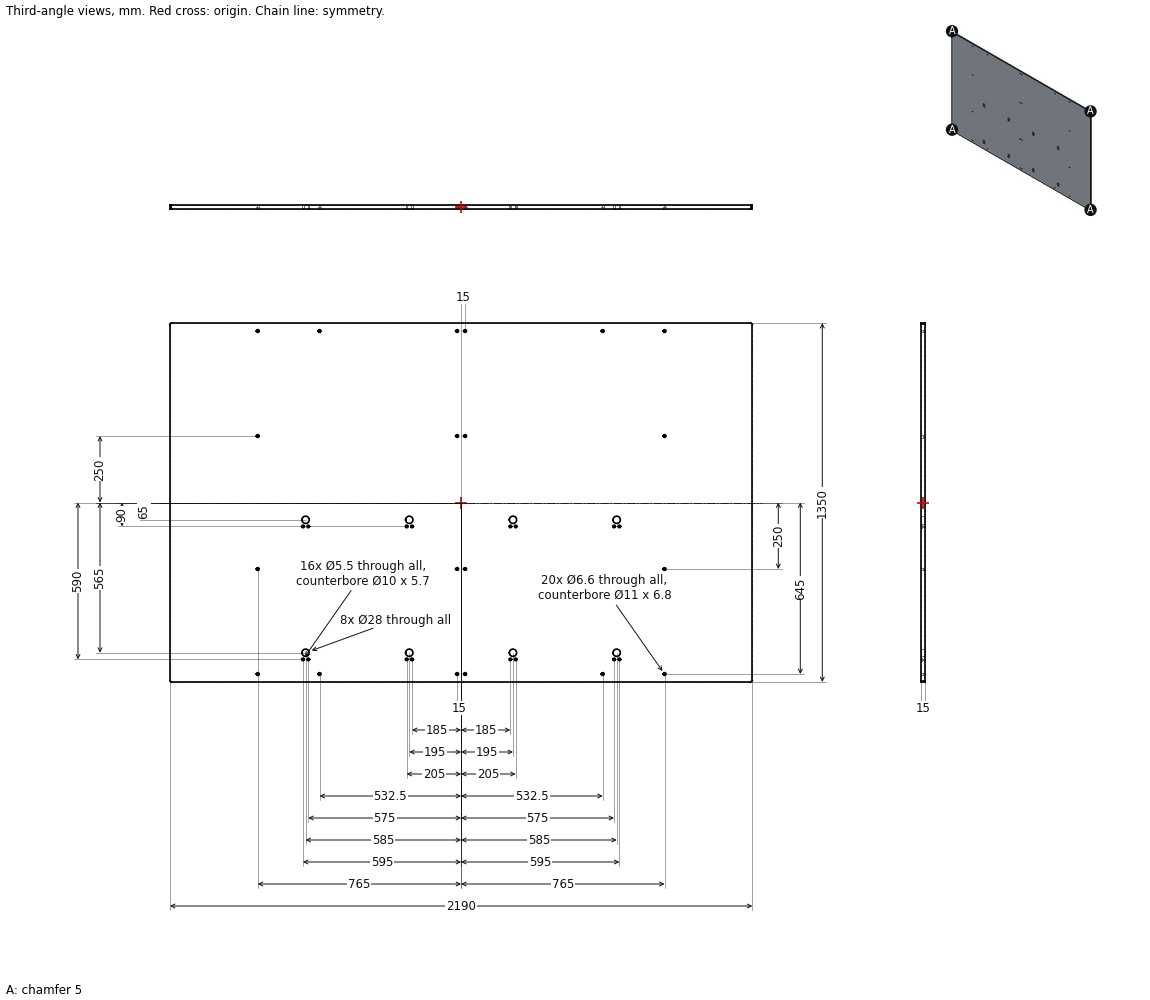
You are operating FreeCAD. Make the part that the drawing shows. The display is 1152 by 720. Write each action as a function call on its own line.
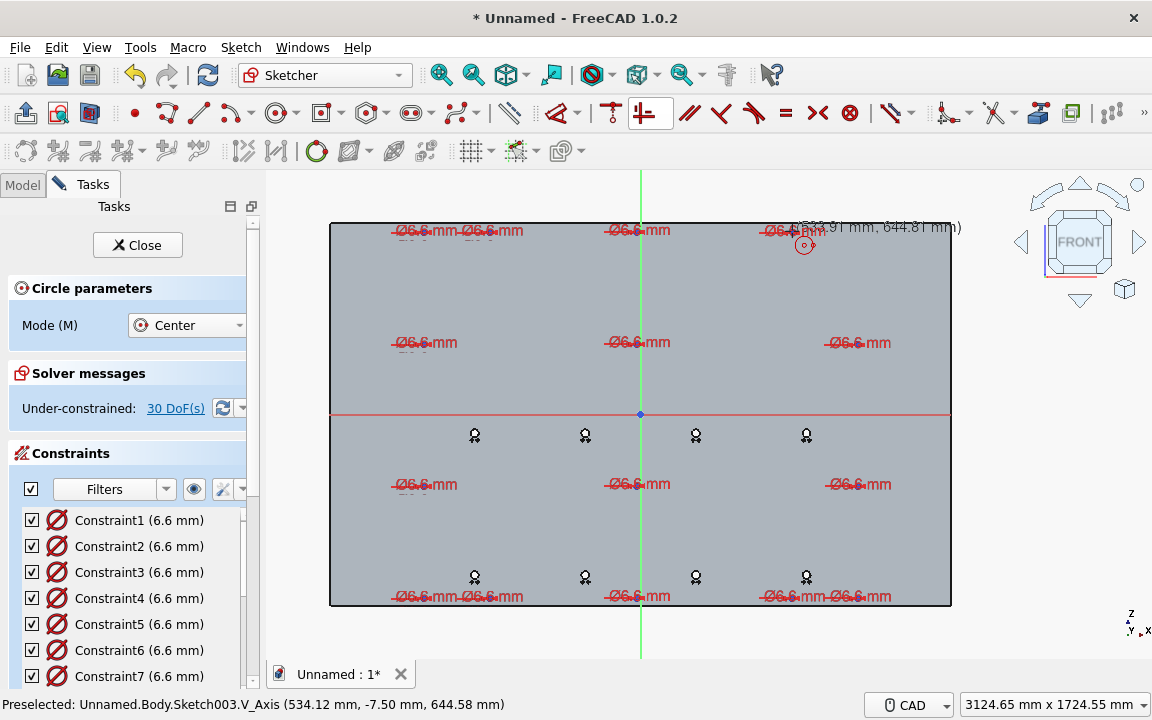
scroll(858, 232, up, 16)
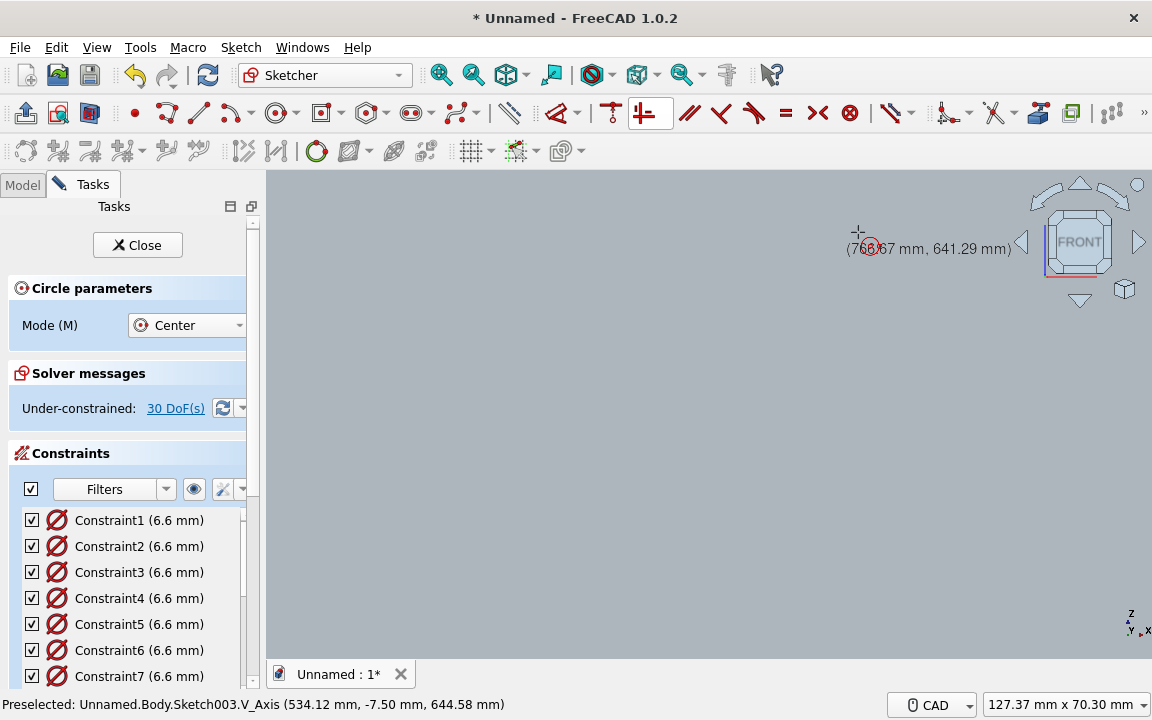
scroll(859, 232, down, 16)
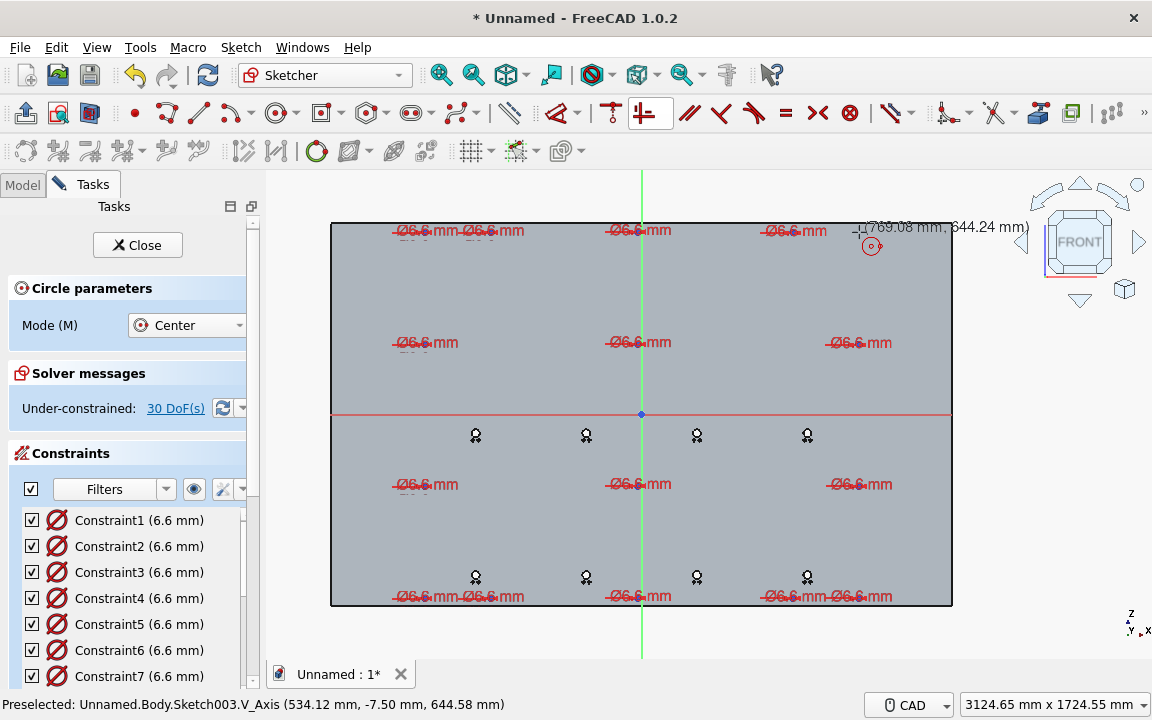
click(858, 232)
move(859, 231)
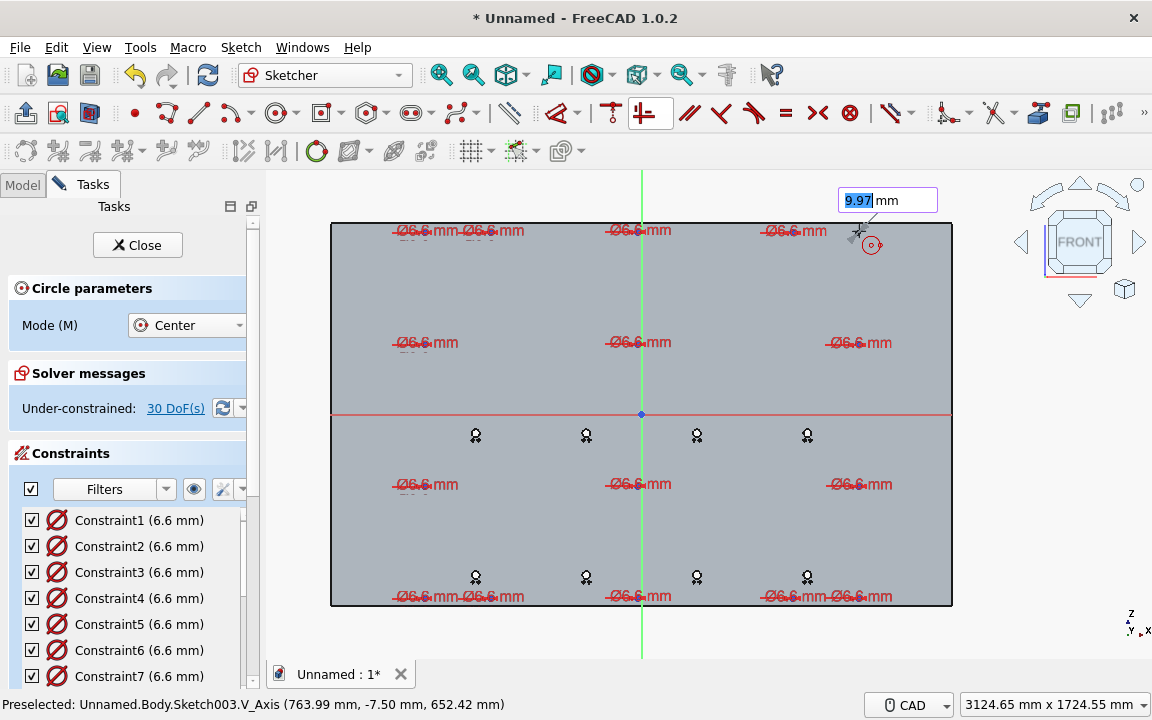
text(6.6)
key(Return)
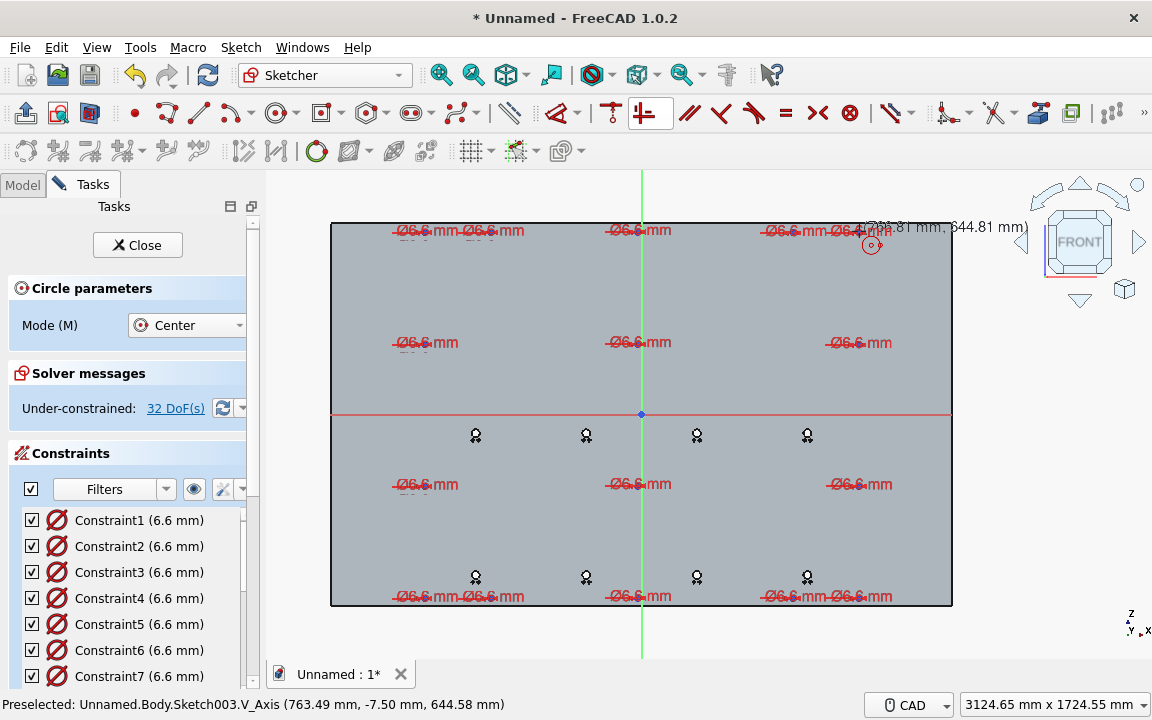
scroll(646, 232, up, 16)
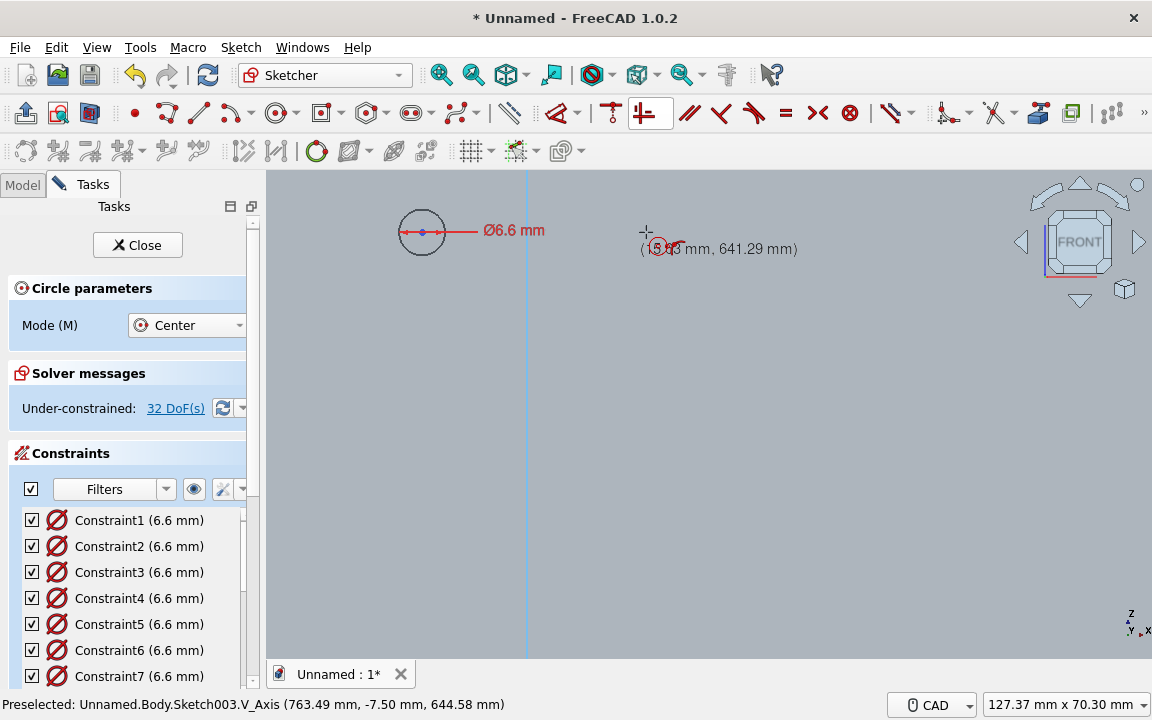
scroll(645, 232, down, 16)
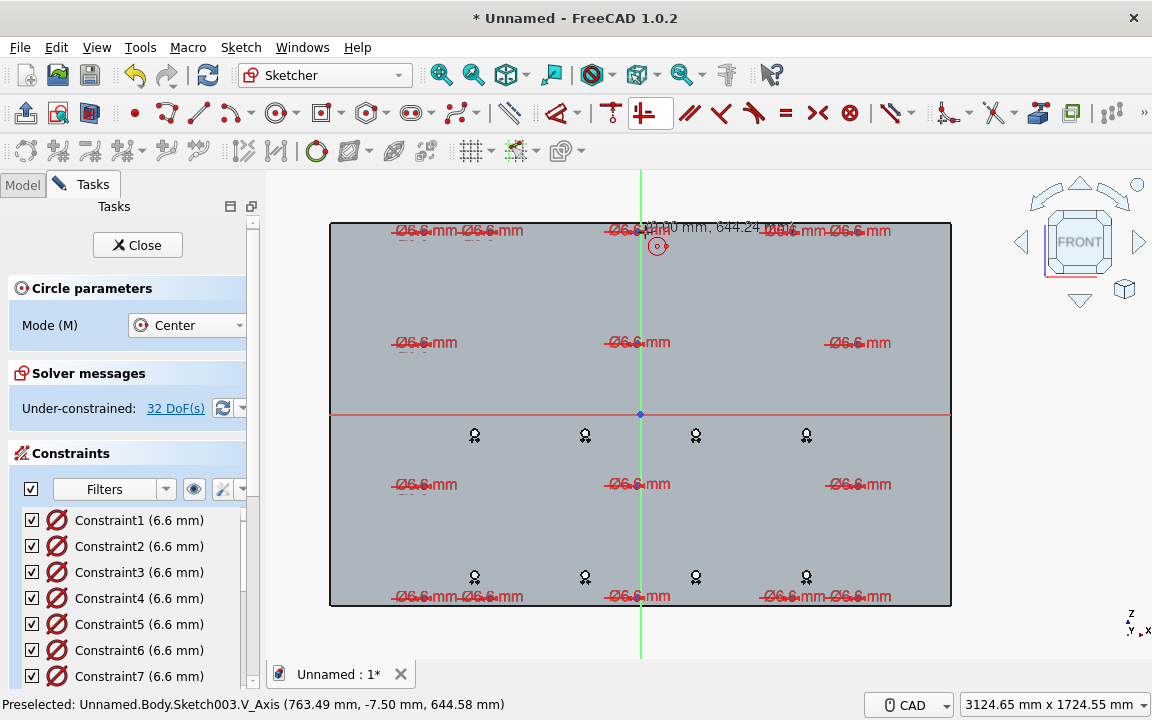
scroll(645, 232, up, 7)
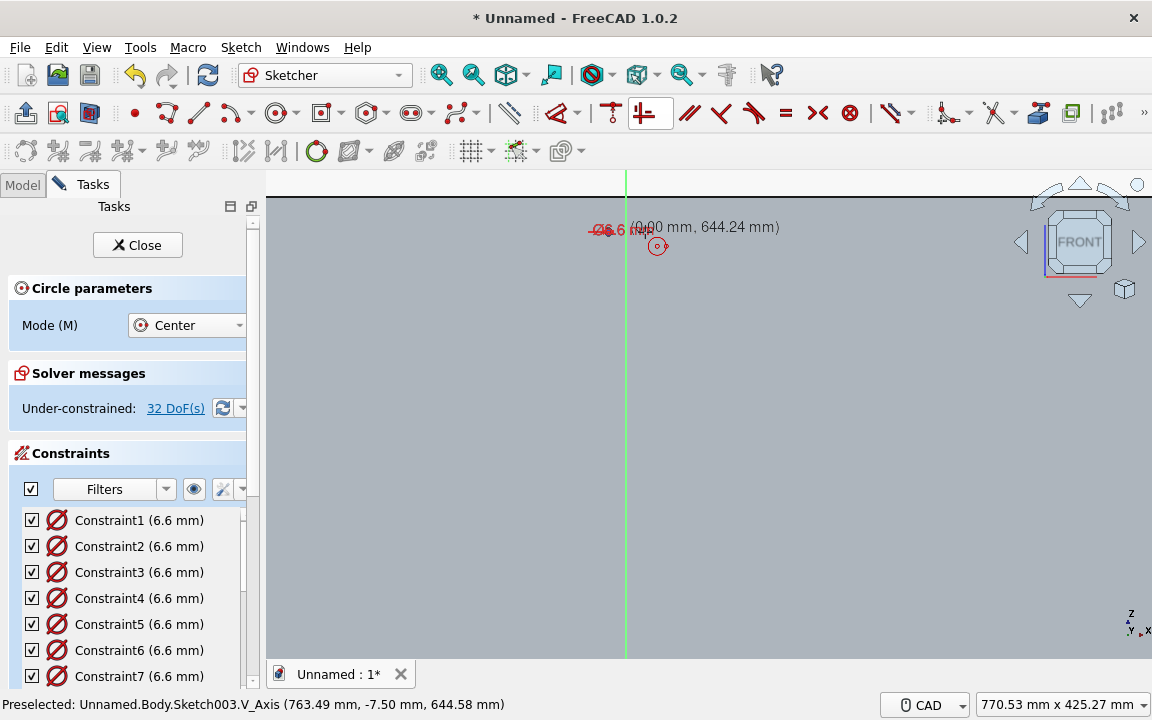
click(643, 231)
move(646, 229)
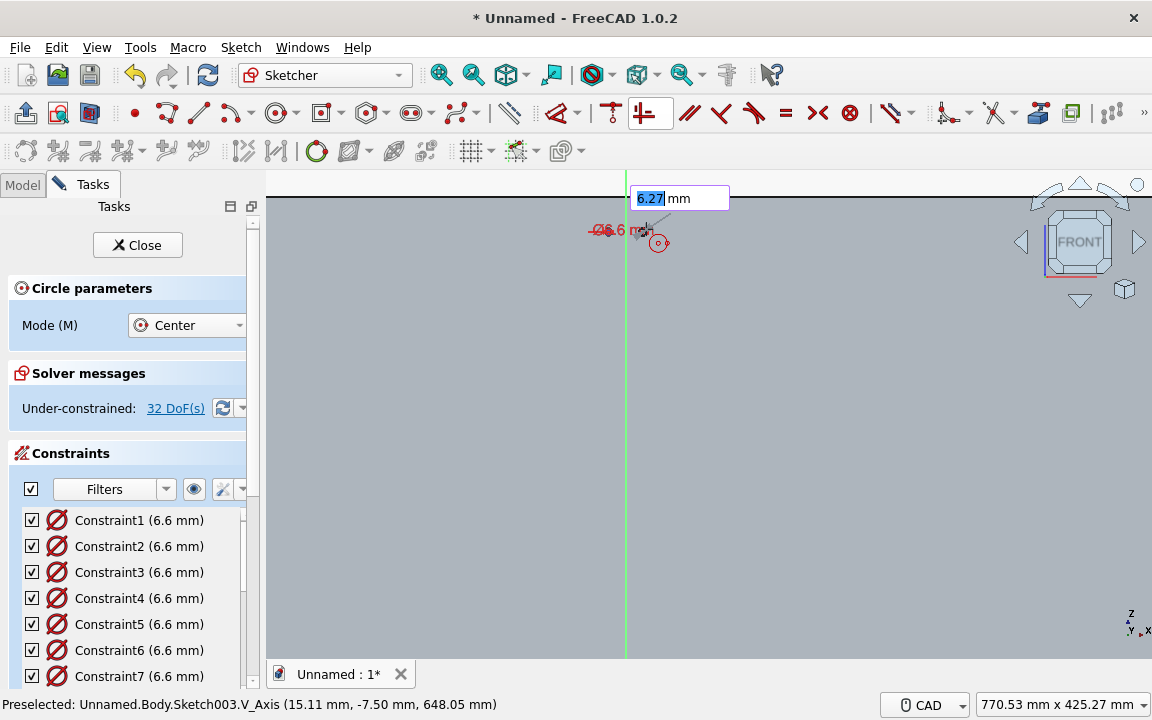
text(6.6)
key(Return)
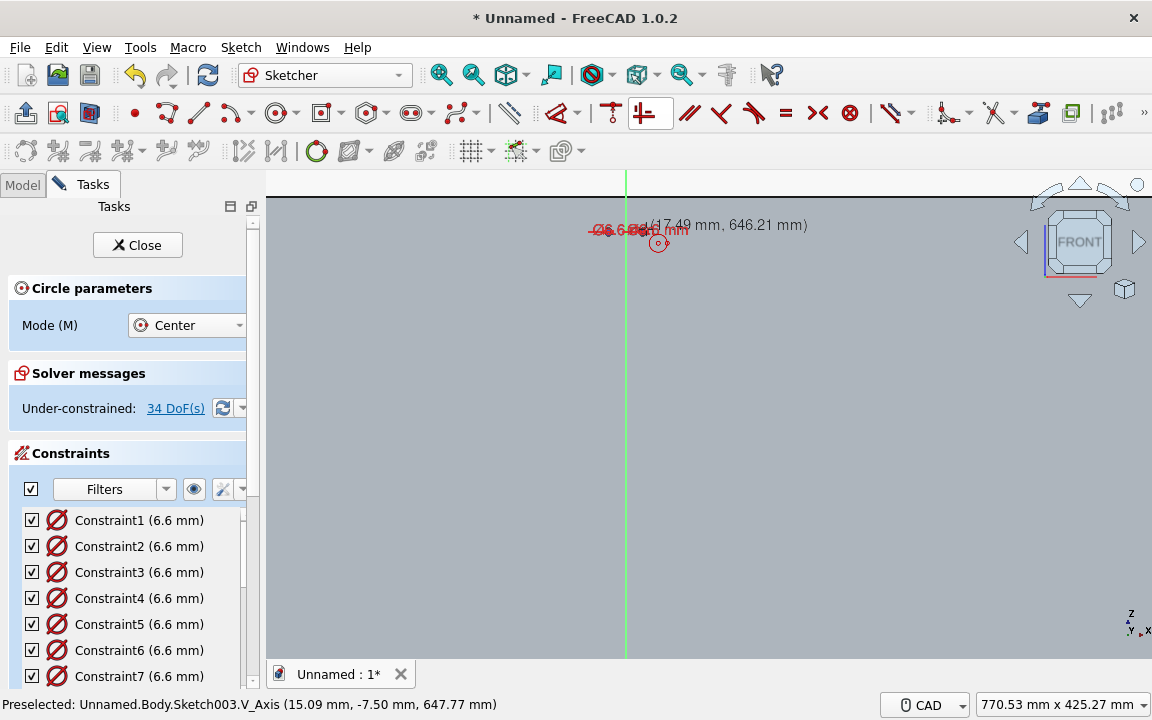
scroll(644, 273, down, 8)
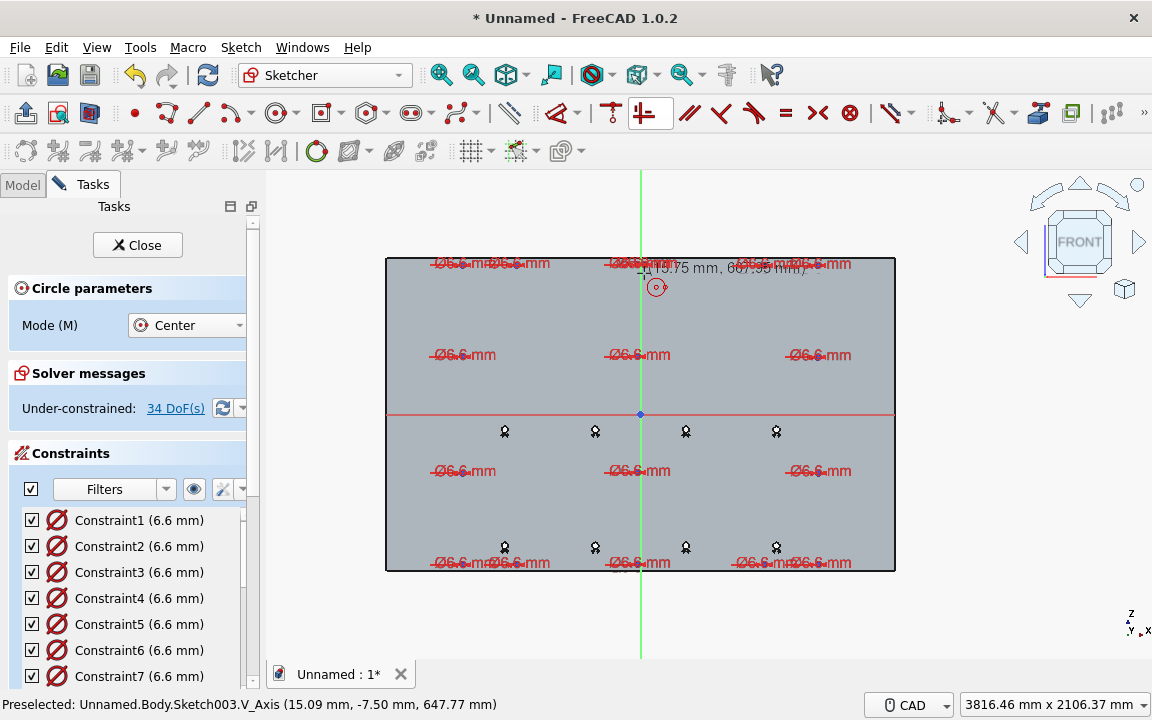
scroll(644, 356, up, 17)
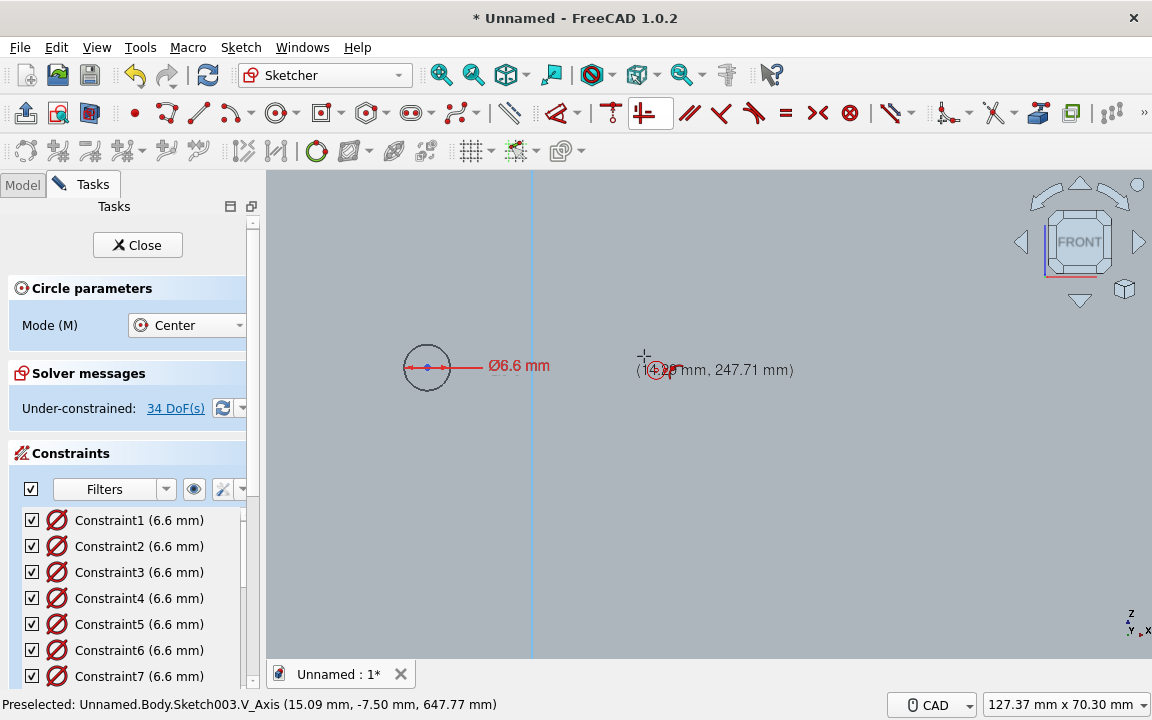
scroll(645, 343, down, 16)